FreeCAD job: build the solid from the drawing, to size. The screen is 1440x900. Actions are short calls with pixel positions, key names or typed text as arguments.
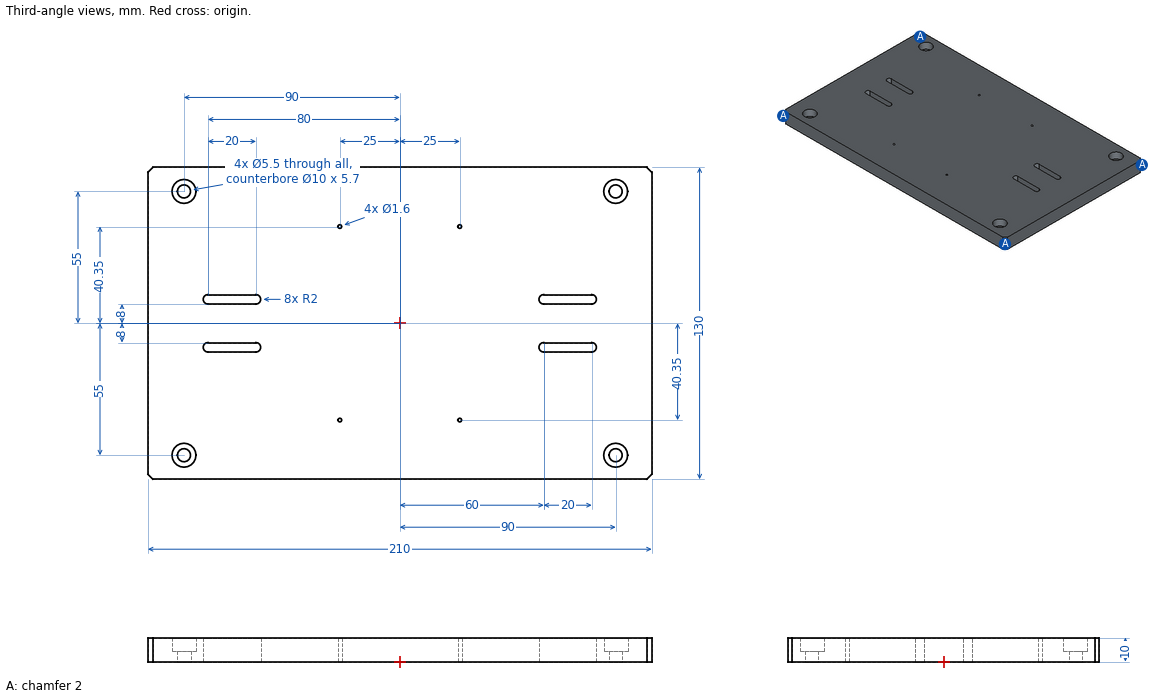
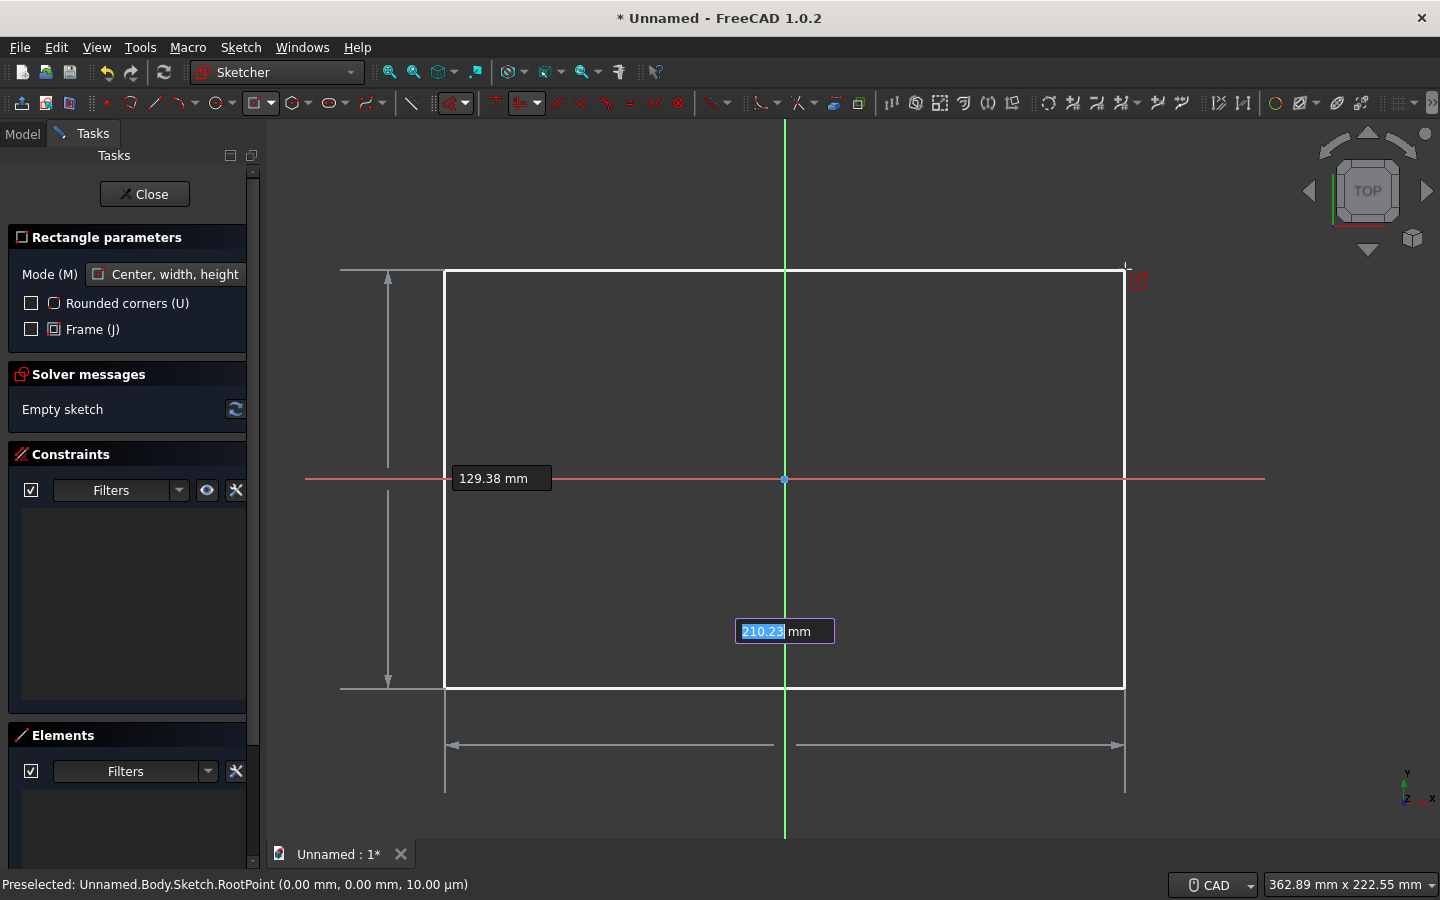
text(210)
key(Tab)
text(130)
key(Return)
key(Escape)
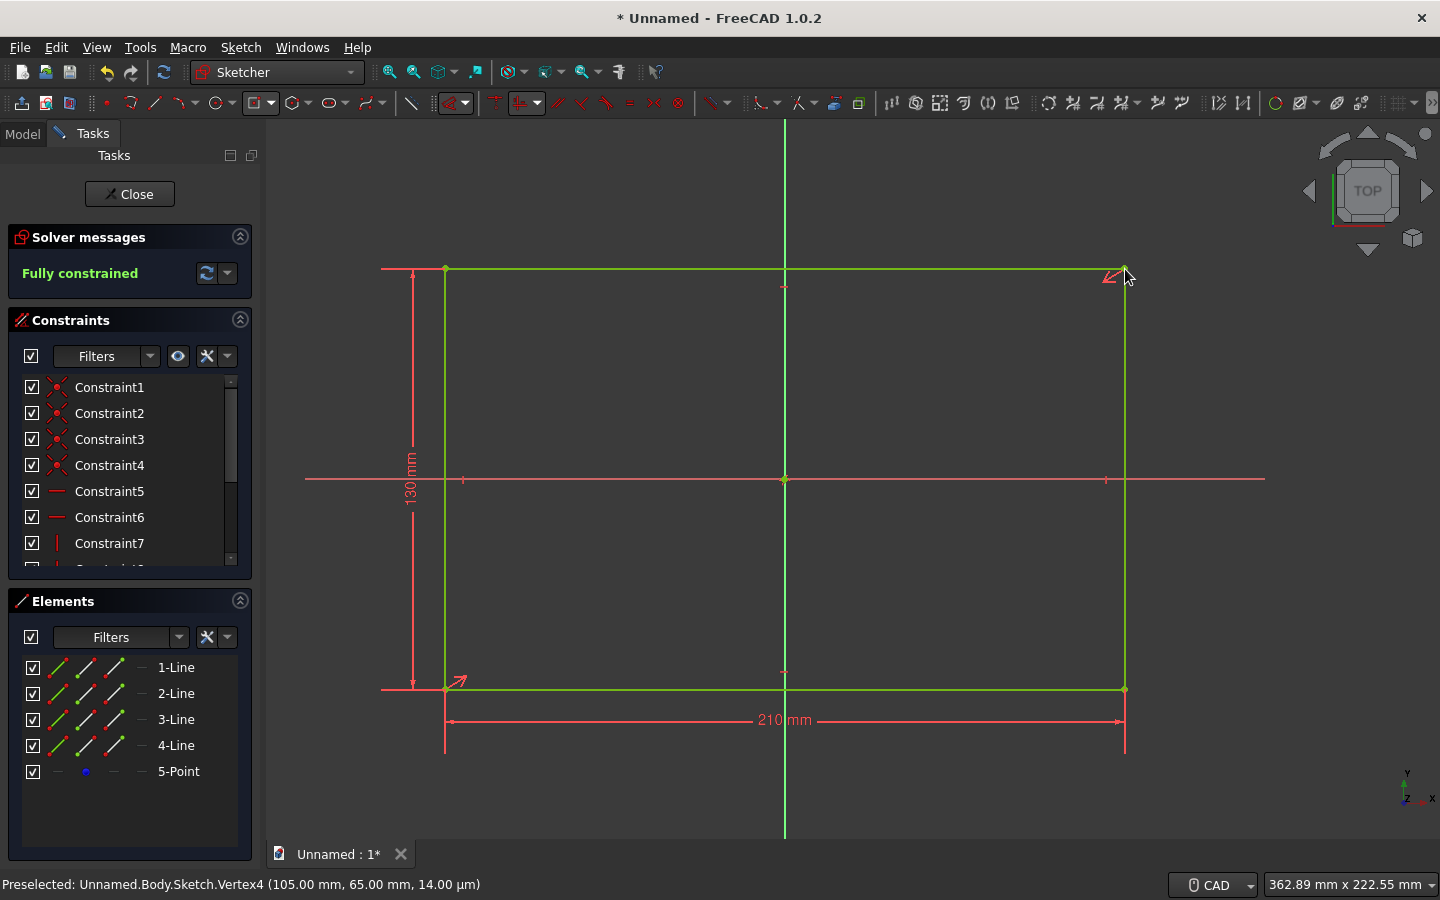
click(130, 194)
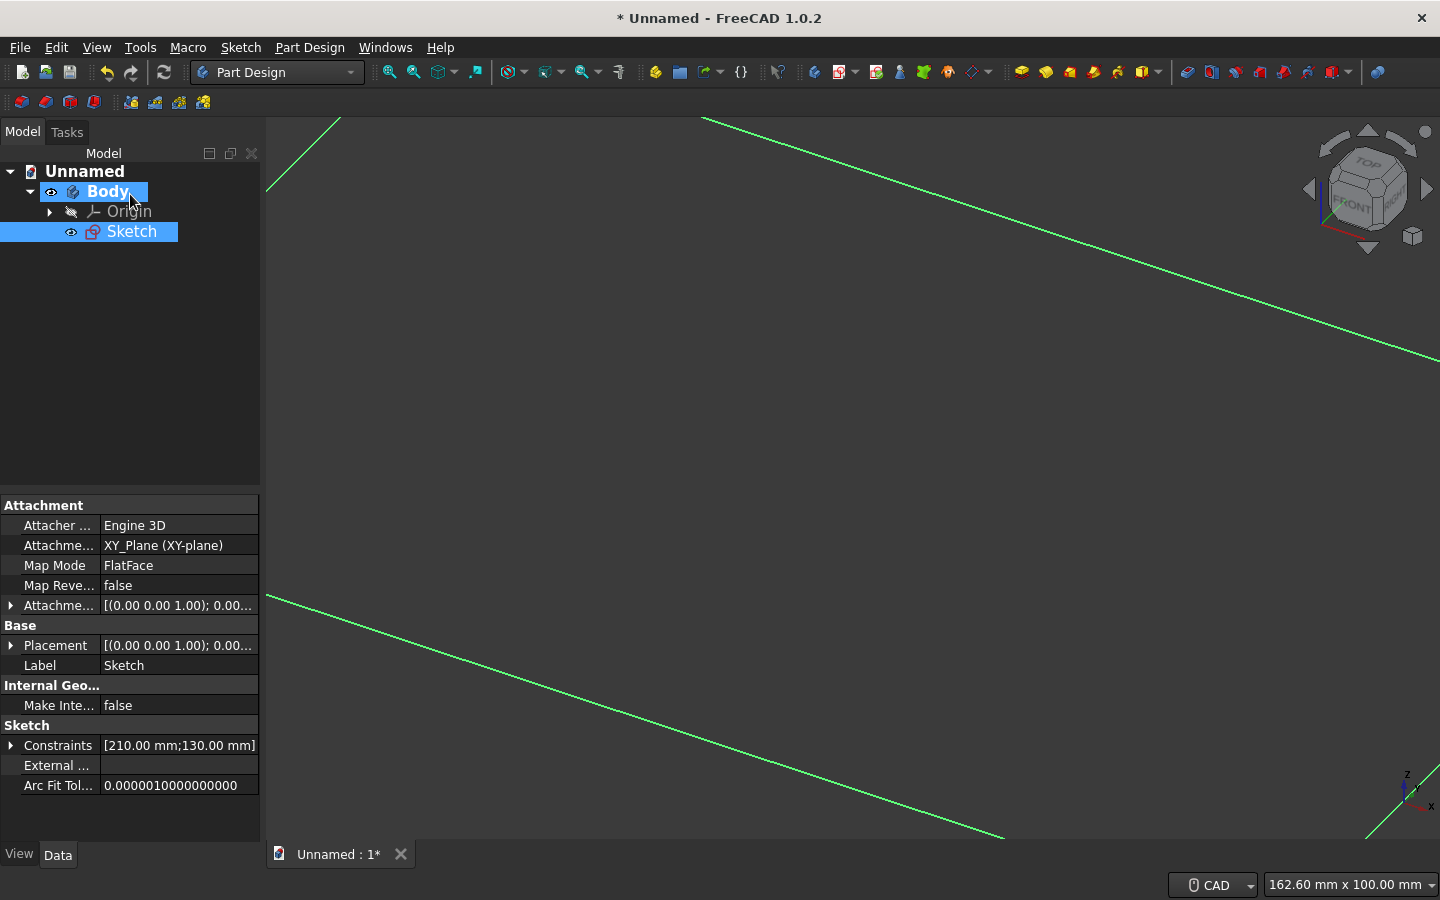
click(1022, 72)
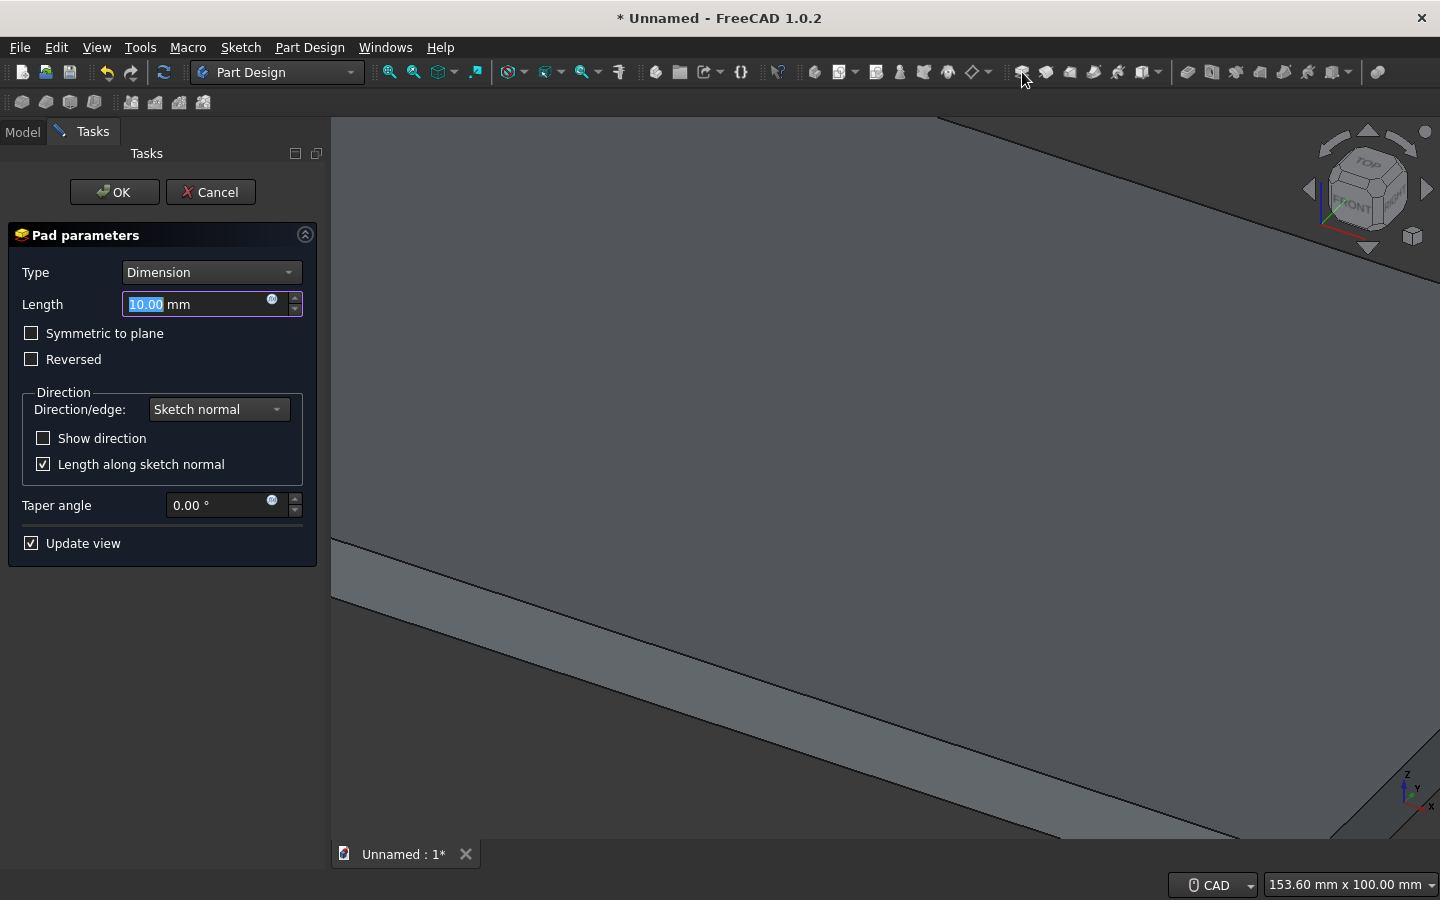
text(10)
key(Tab)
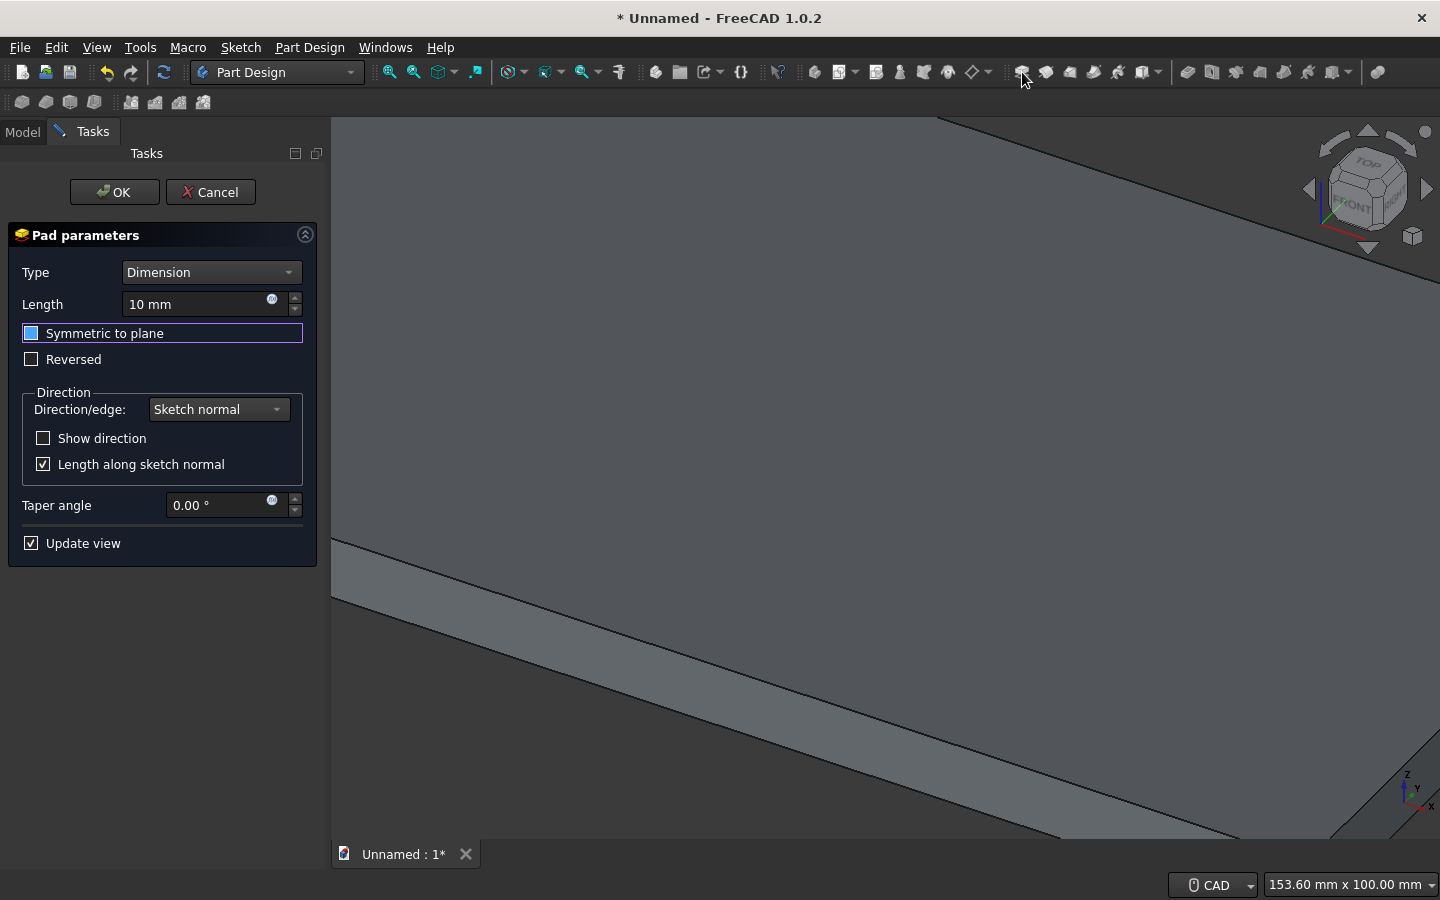
click(115, 192)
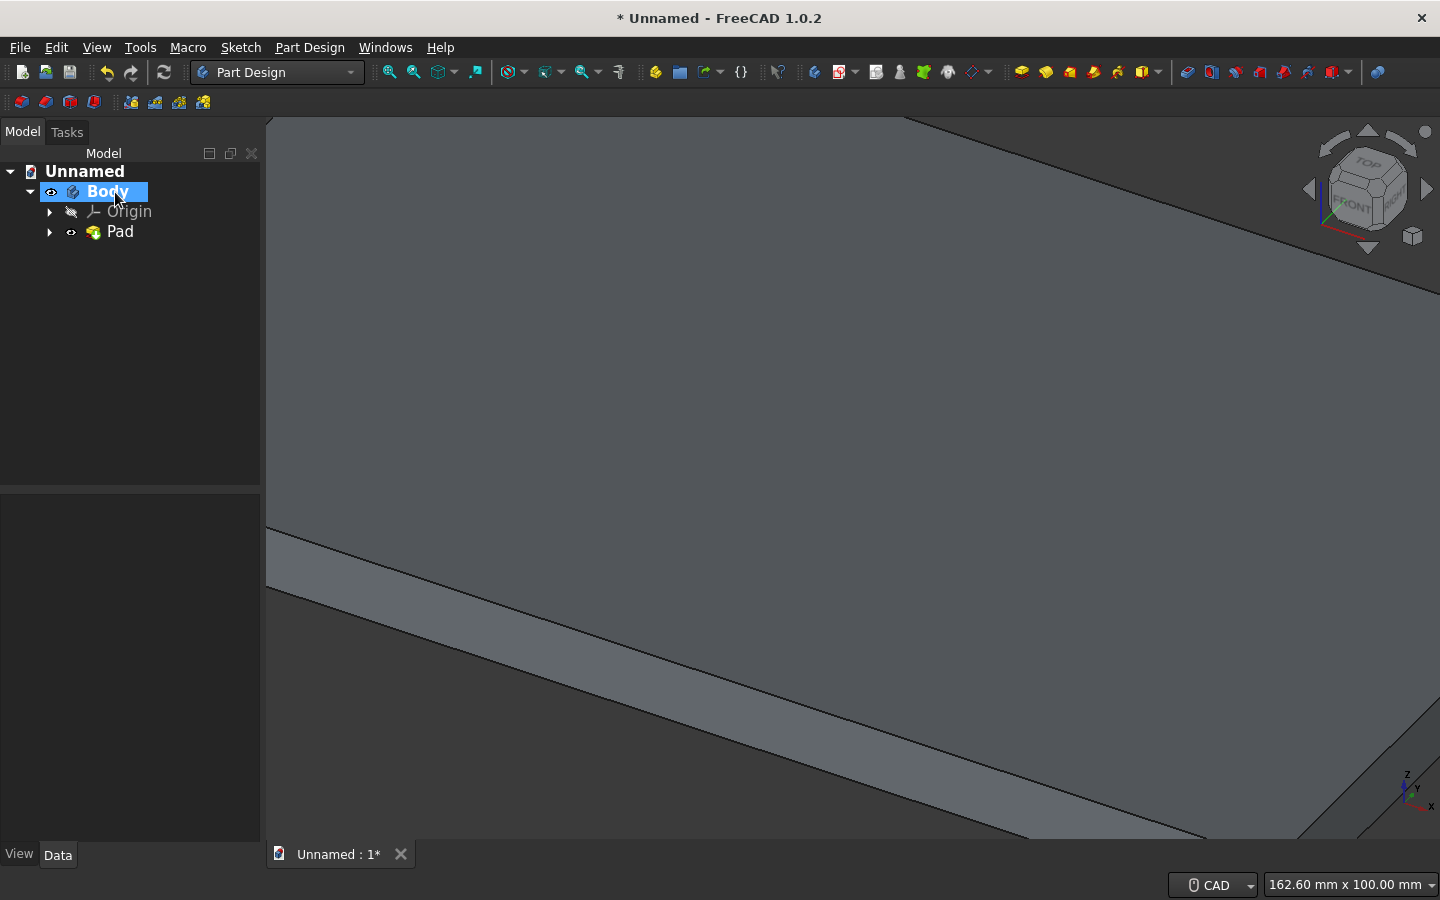
click(390, 72)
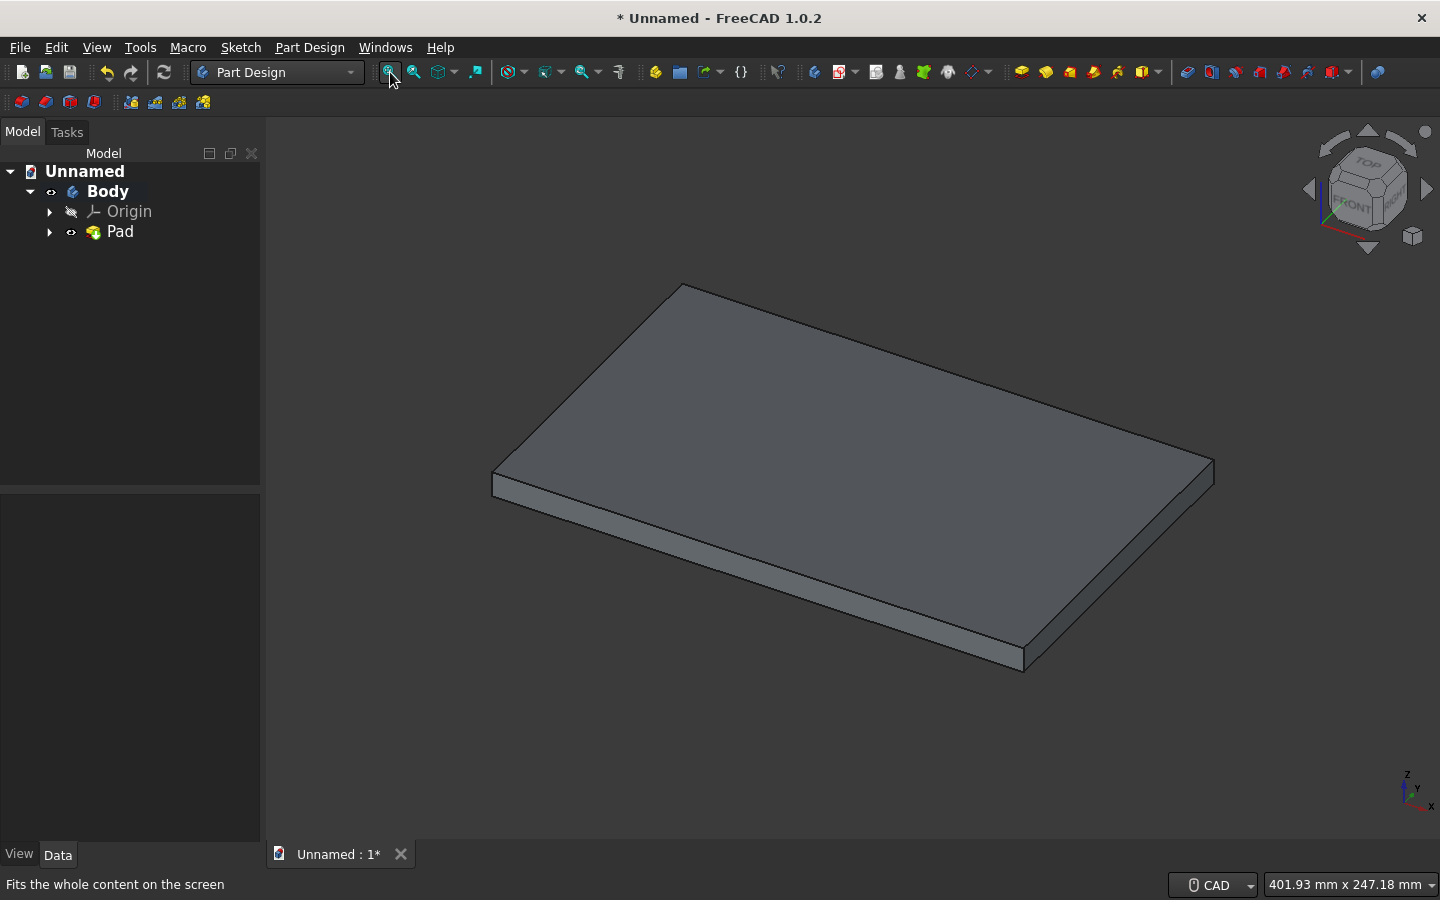
click(929, 490)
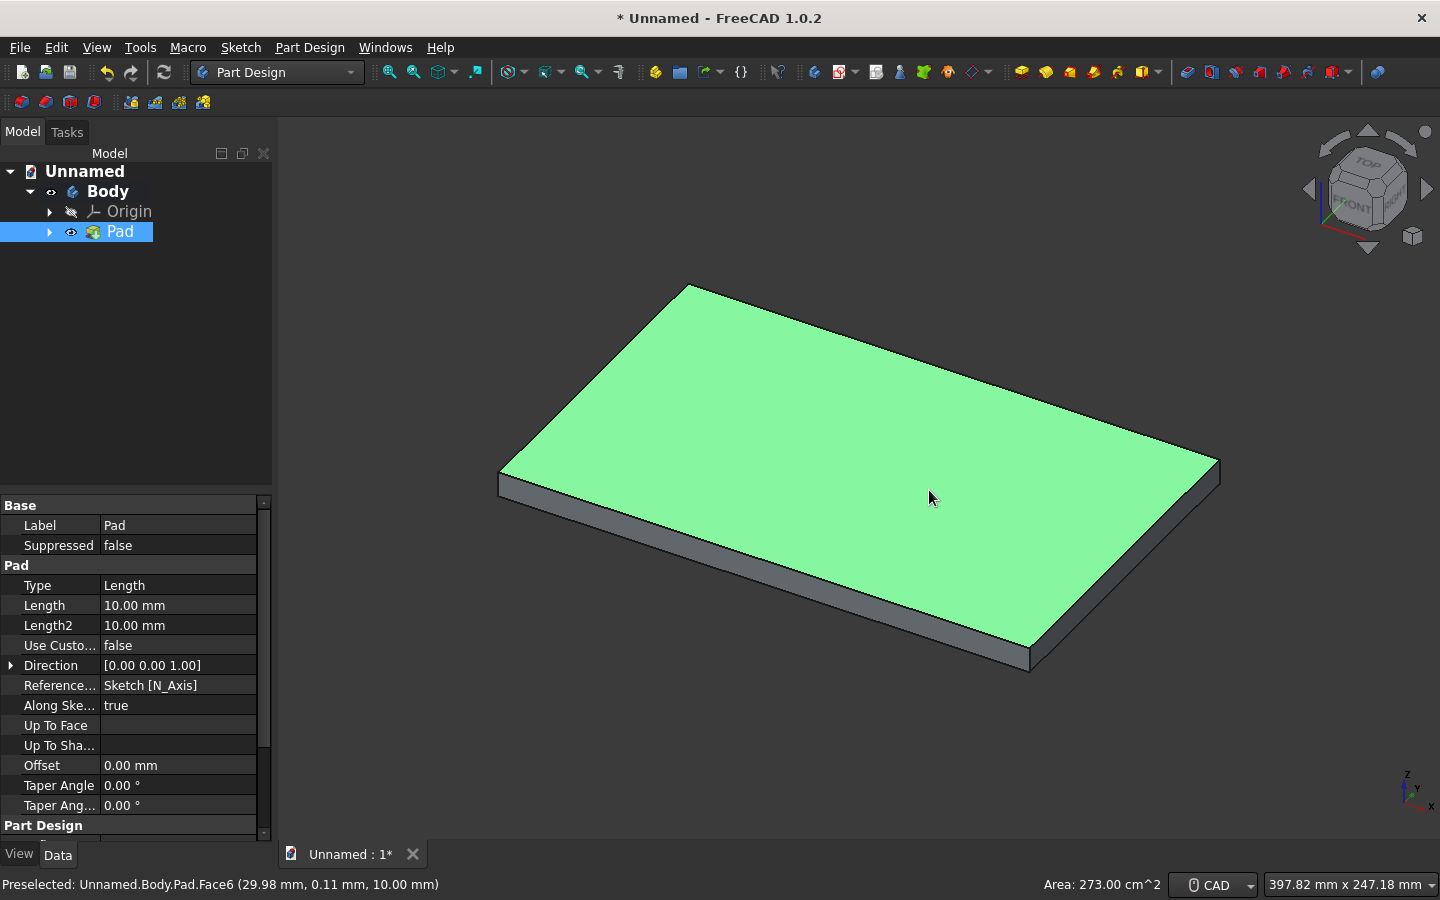
click(840, 72)